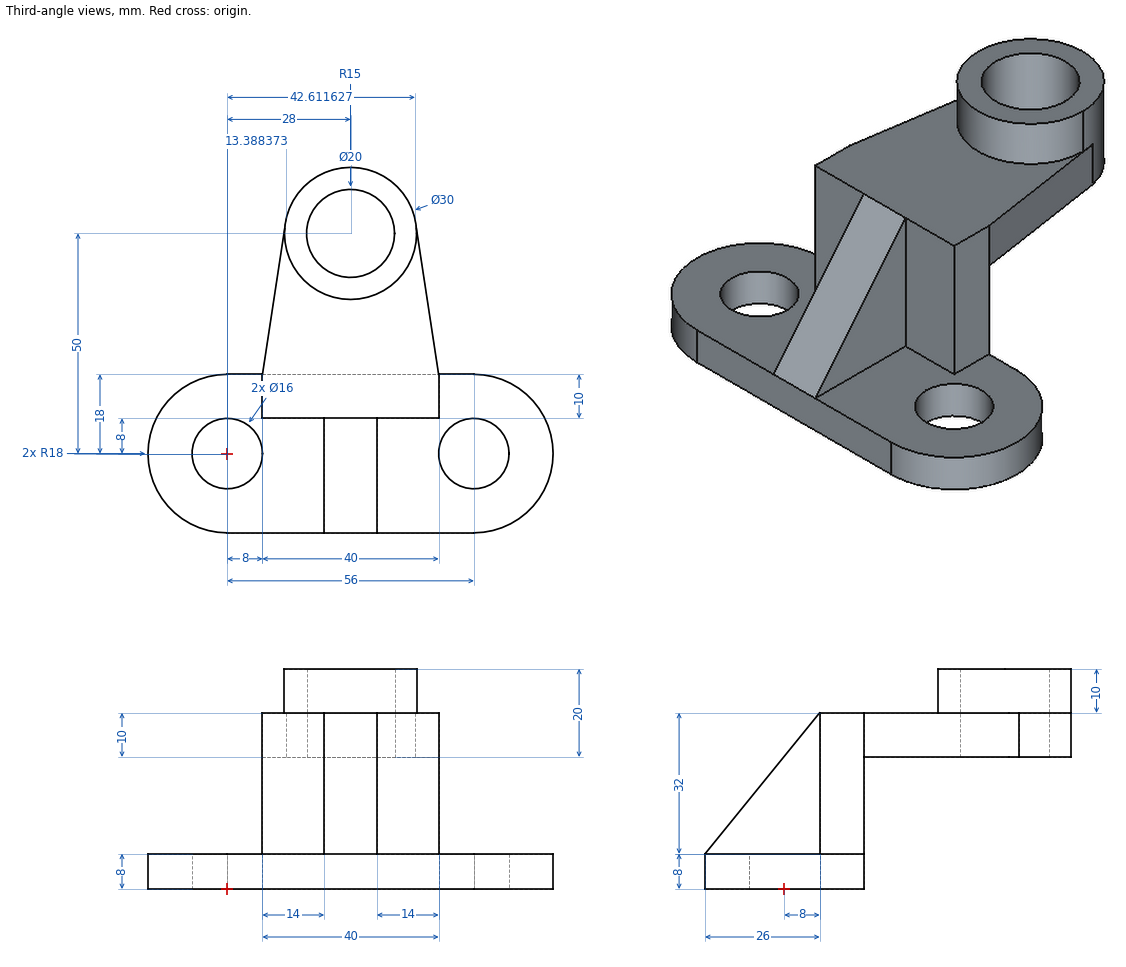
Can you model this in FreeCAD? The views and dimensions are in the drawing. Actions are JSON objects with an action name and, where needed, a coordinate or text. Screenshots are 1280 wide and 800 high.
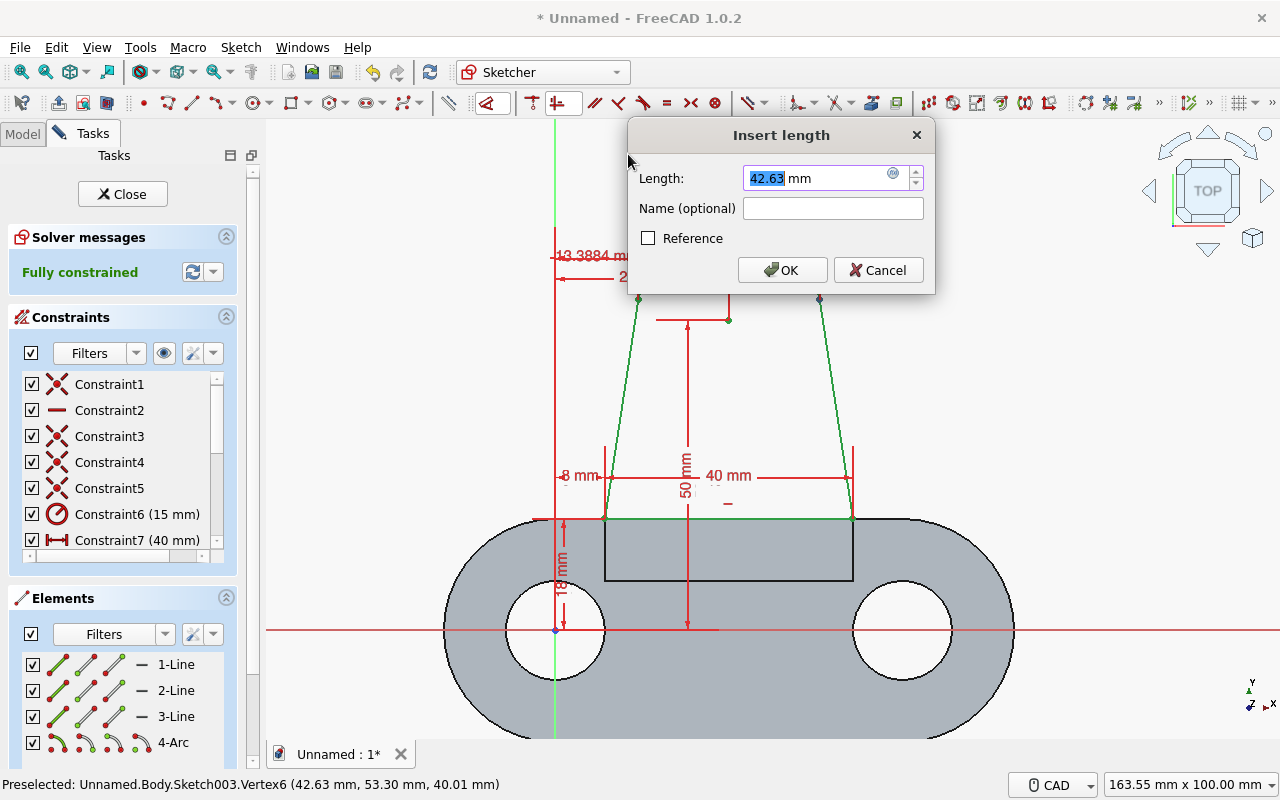
{"action": "type", "text": "42.611627"}
{"action": "key", "text": "Return"}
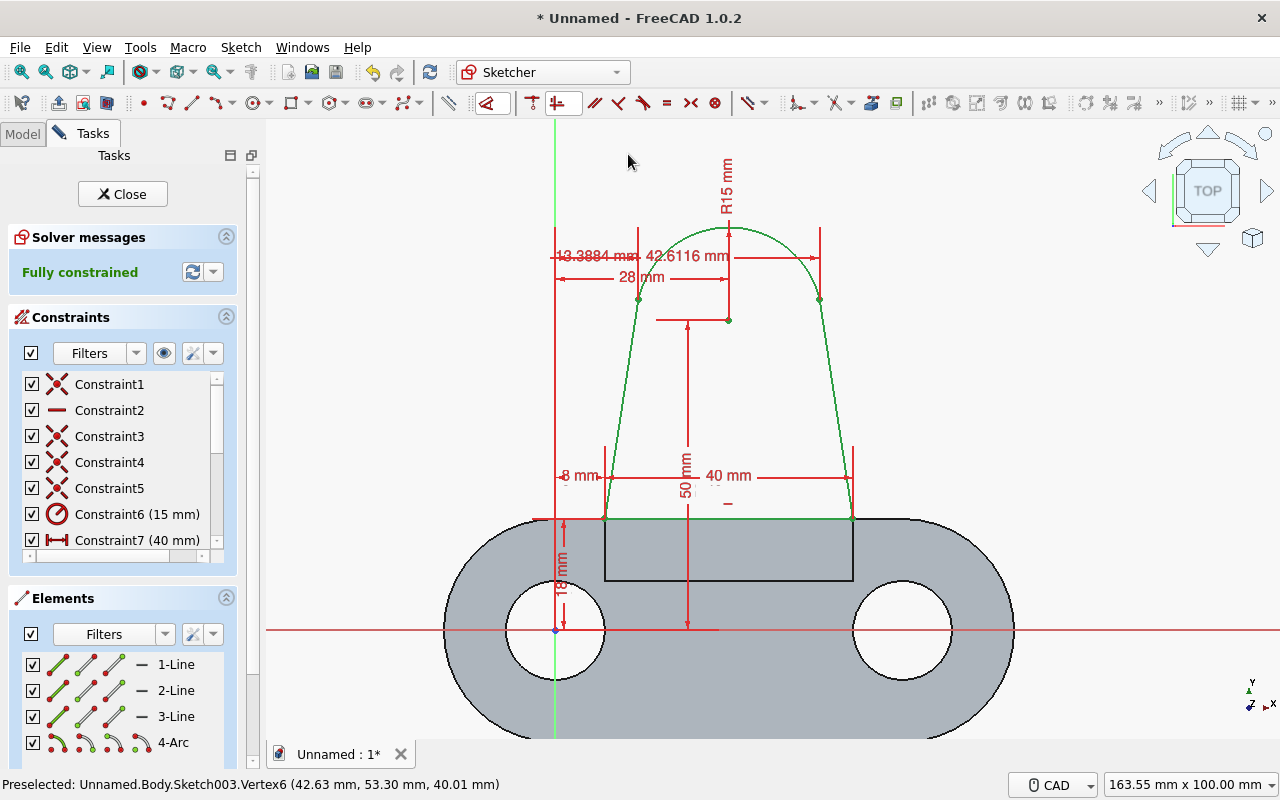
{"action": "left_click", "coordinate": [123, 194]}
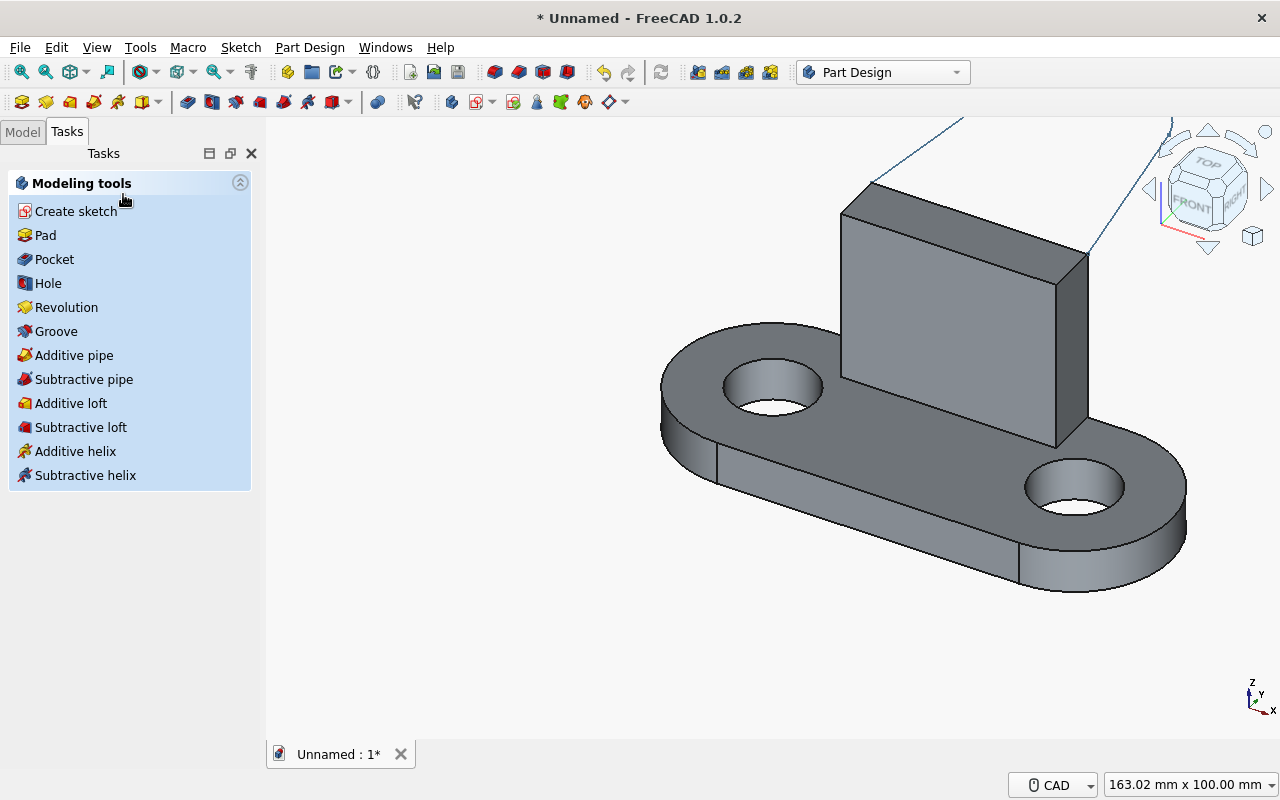
{"action": "left_click", "coordinate": [22, 102]}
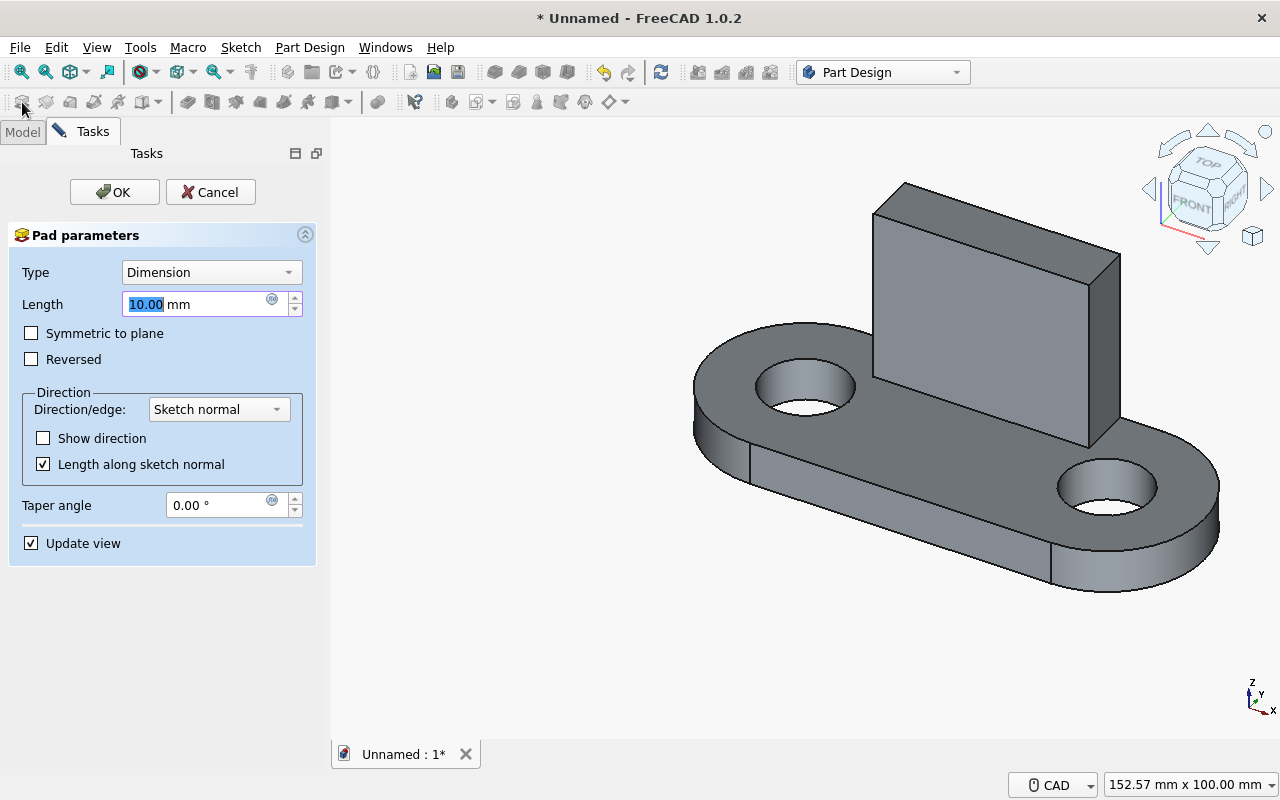
{"action": "type", "text": "10"}
{"action": "key", "text": "Tab"}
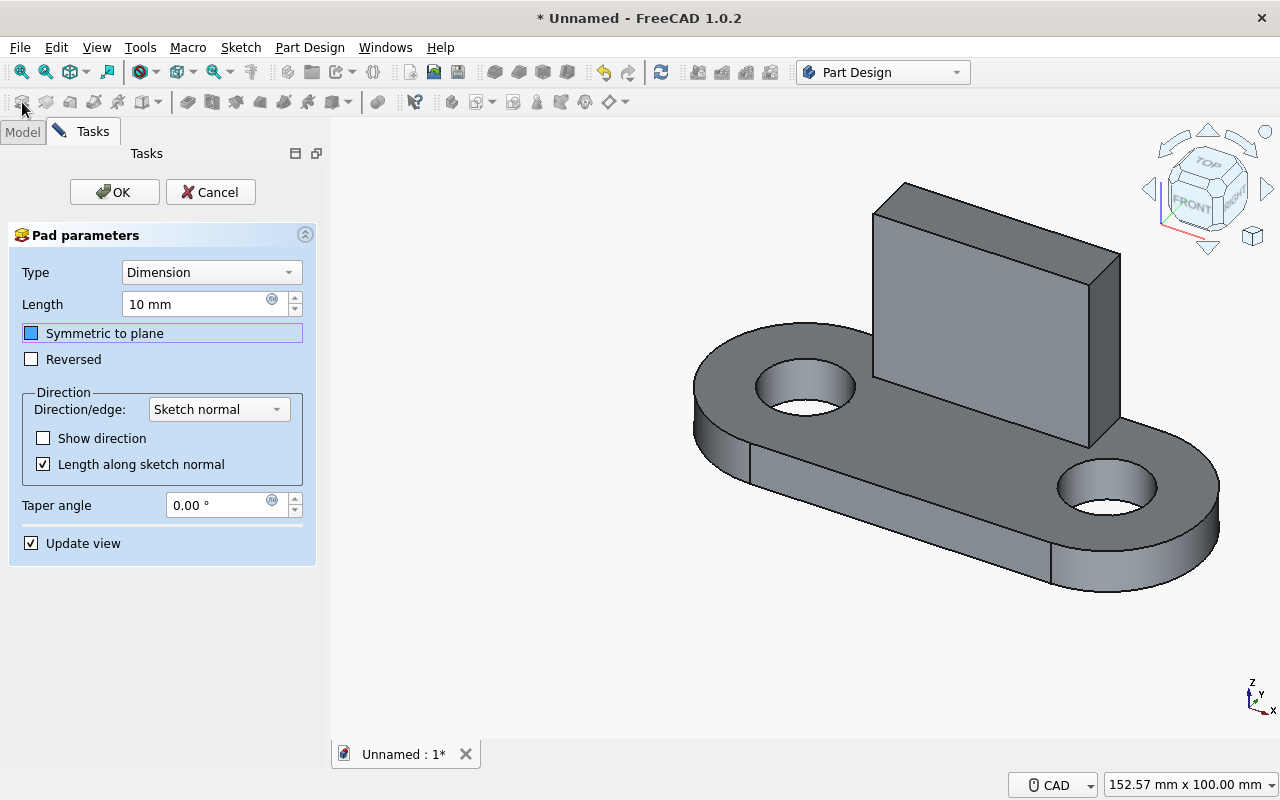
{"action": "left_click", "coordinate": [30, 359]}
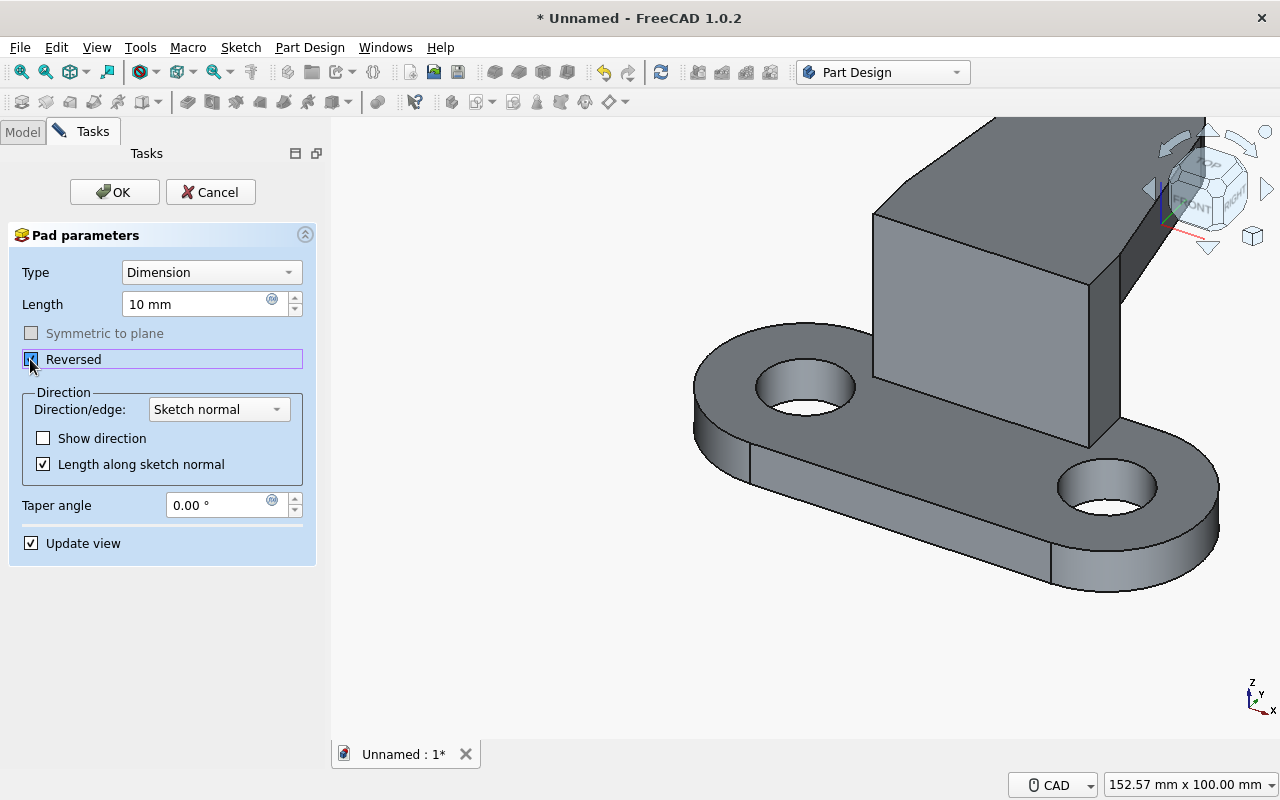
{"action": "left_click", "coordinate": [115, 192]}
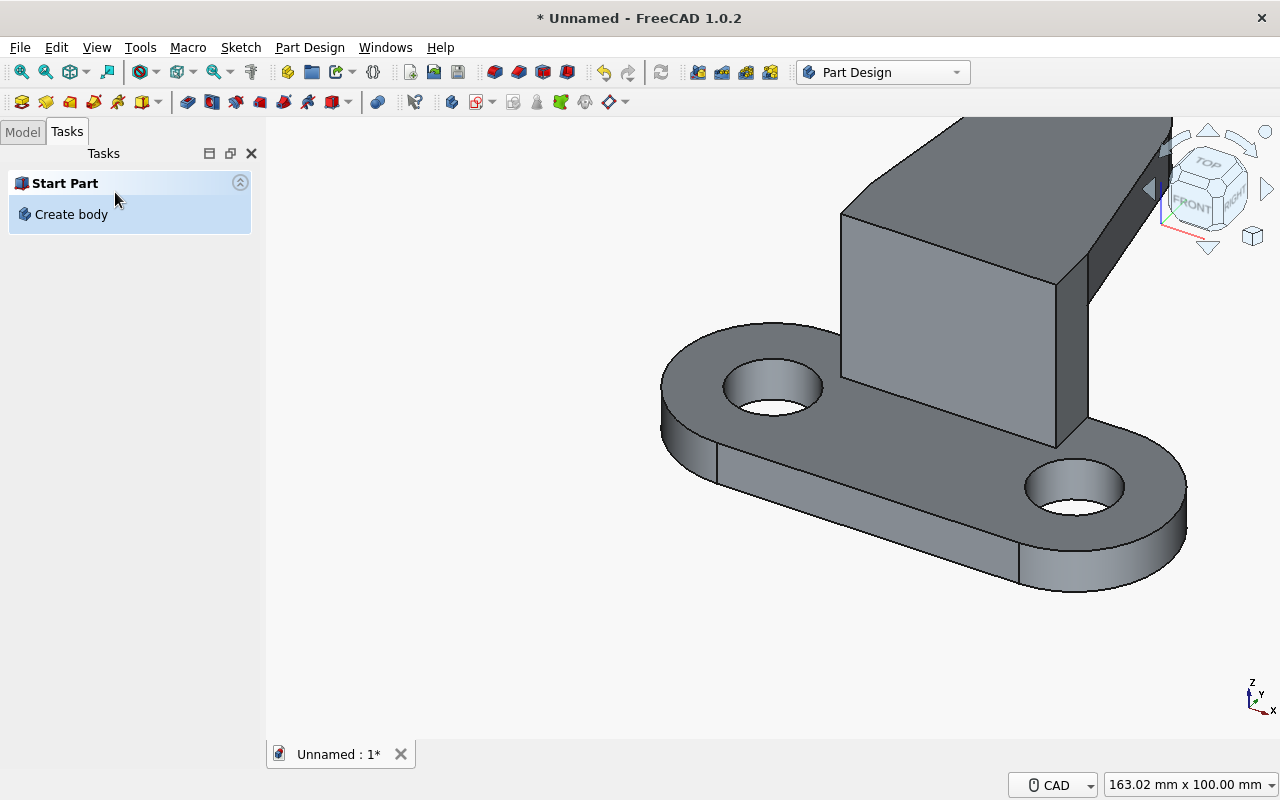
{"action": "left_click", "coordinate": [22, 72]}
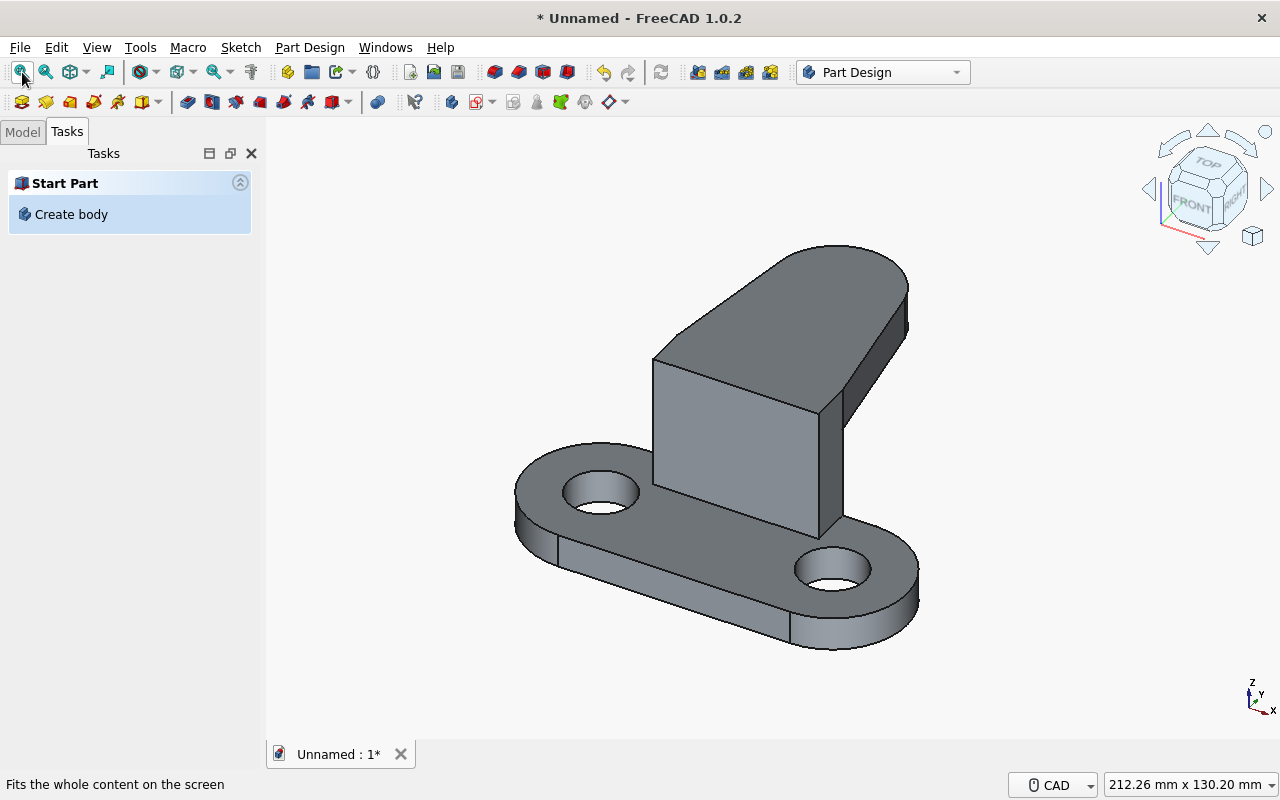
{"action": "left_click", "coordinate": [23, 131]}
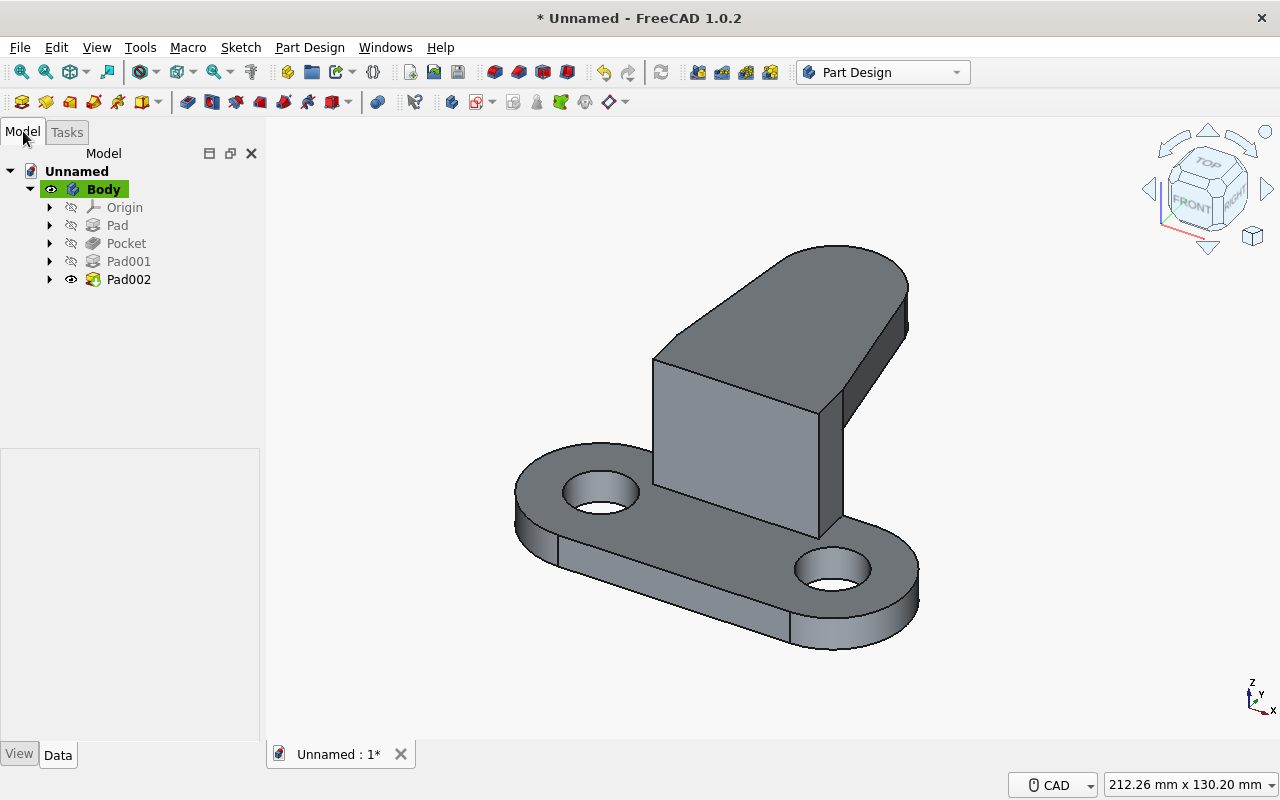
{"action": "left_click", "coordinate": [50, 207]}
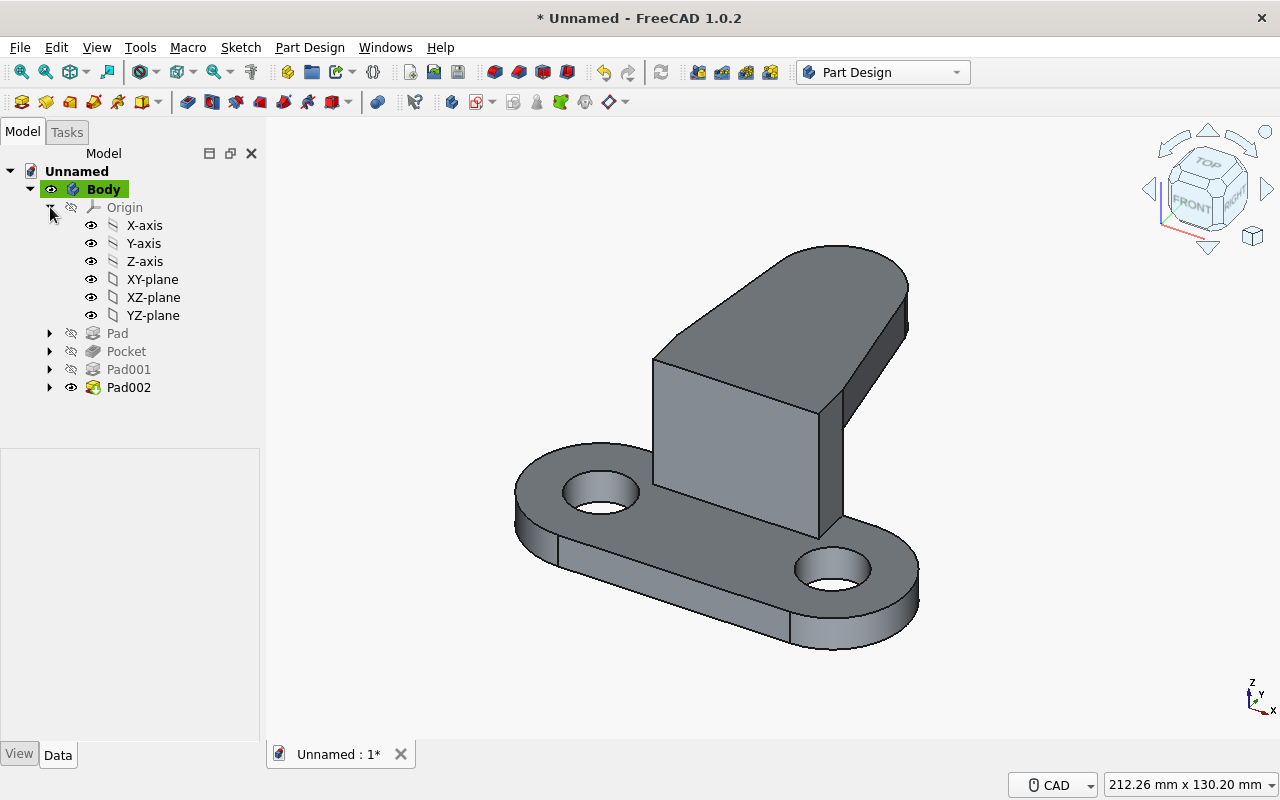
{"action": "left_click", "coordinate": [136, 279]}